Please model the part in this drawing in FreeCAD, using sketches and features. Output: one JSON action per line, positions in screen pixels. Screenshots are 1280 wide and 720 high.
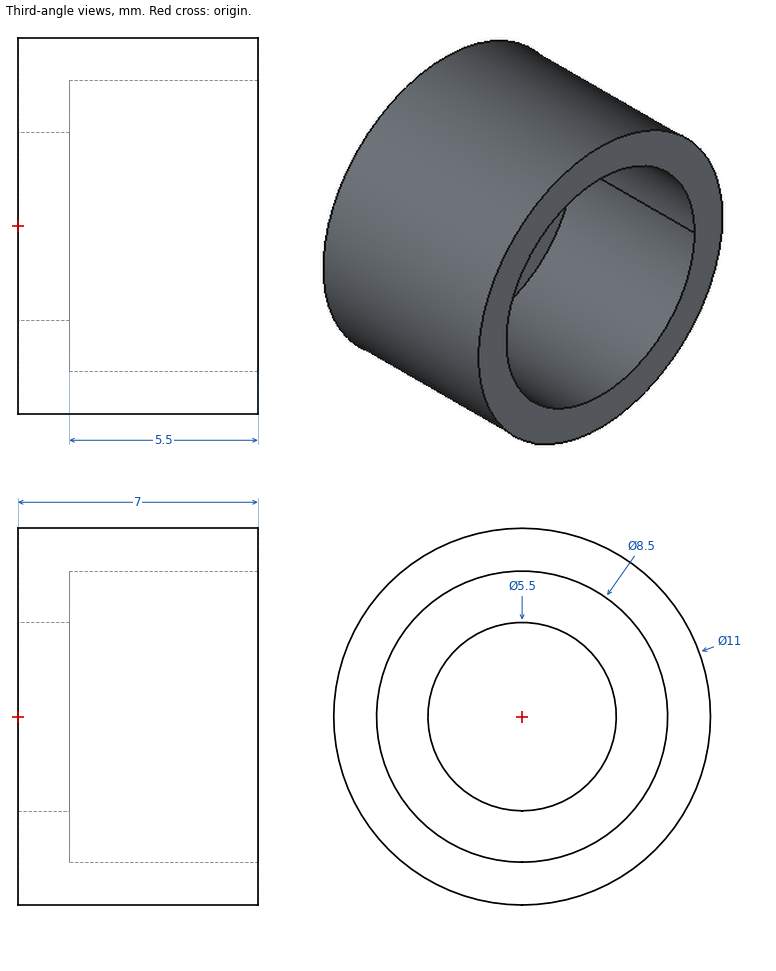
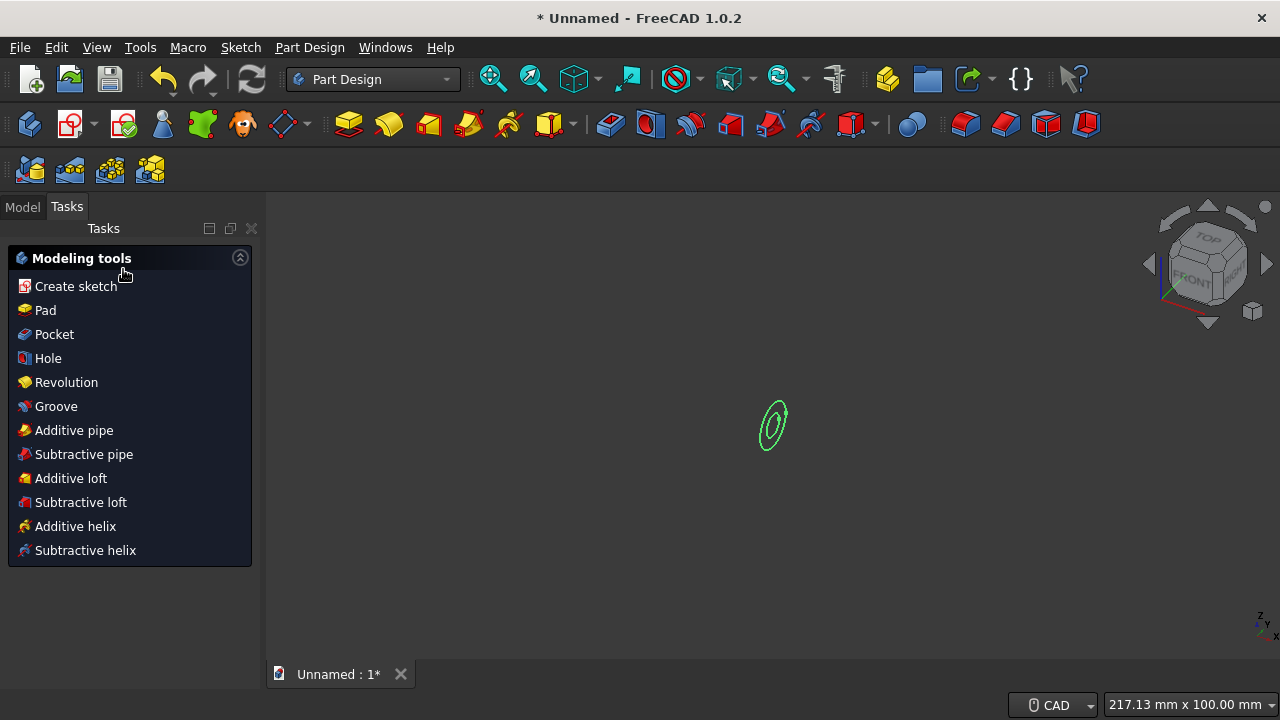
{"action": "left_click", "coordinate": [350, 124]}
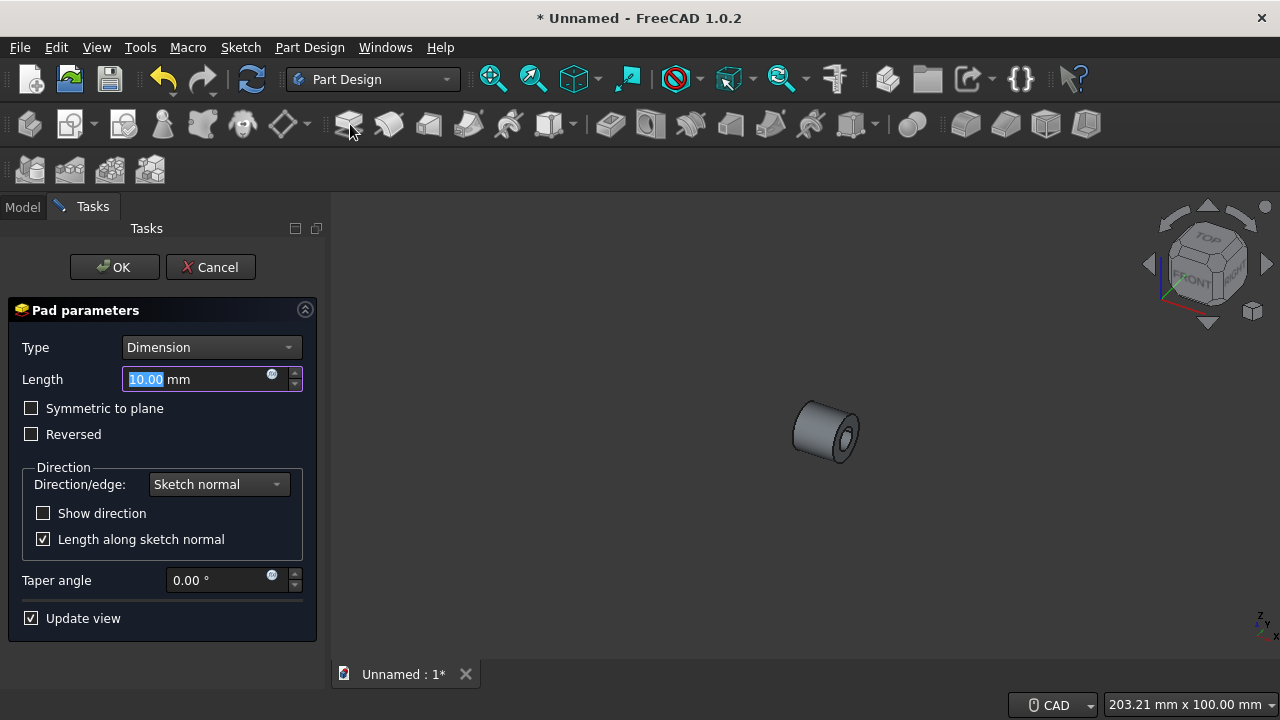
{"action": "type", "text": "7"}
{"action": "key", "text": "Tab"}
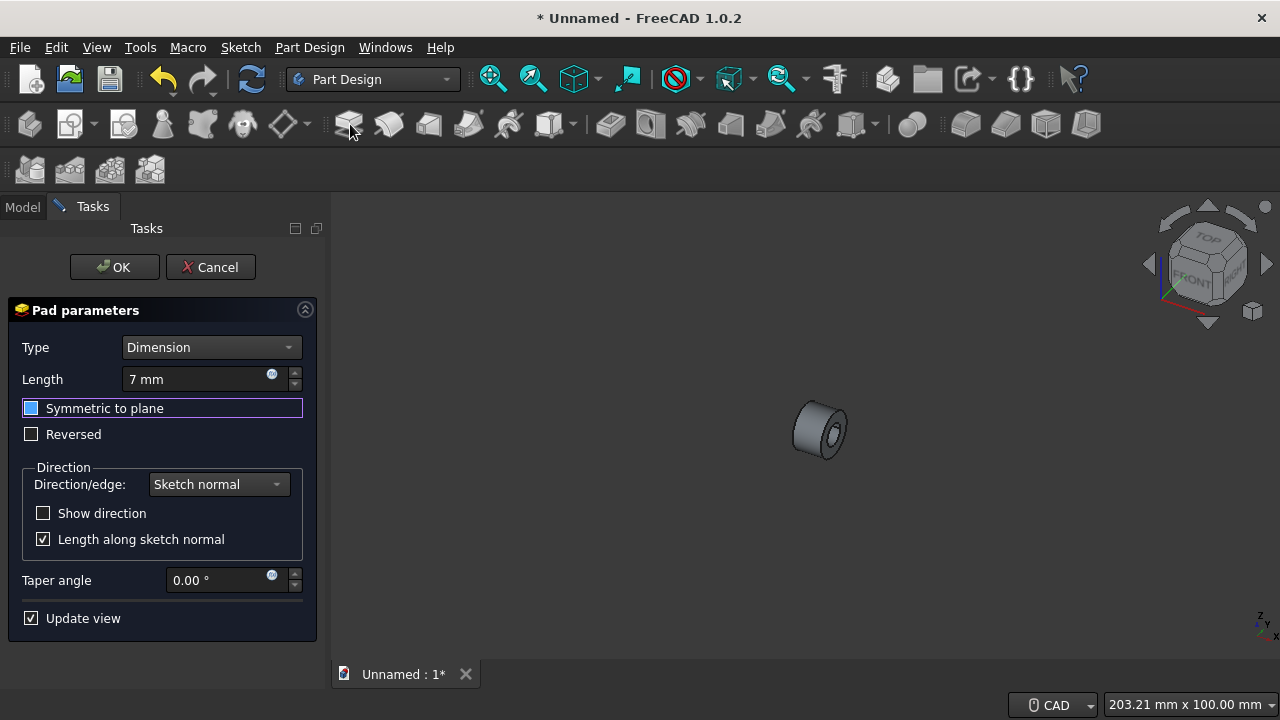
{"action": "left_click", "coordinate": [115, 267]}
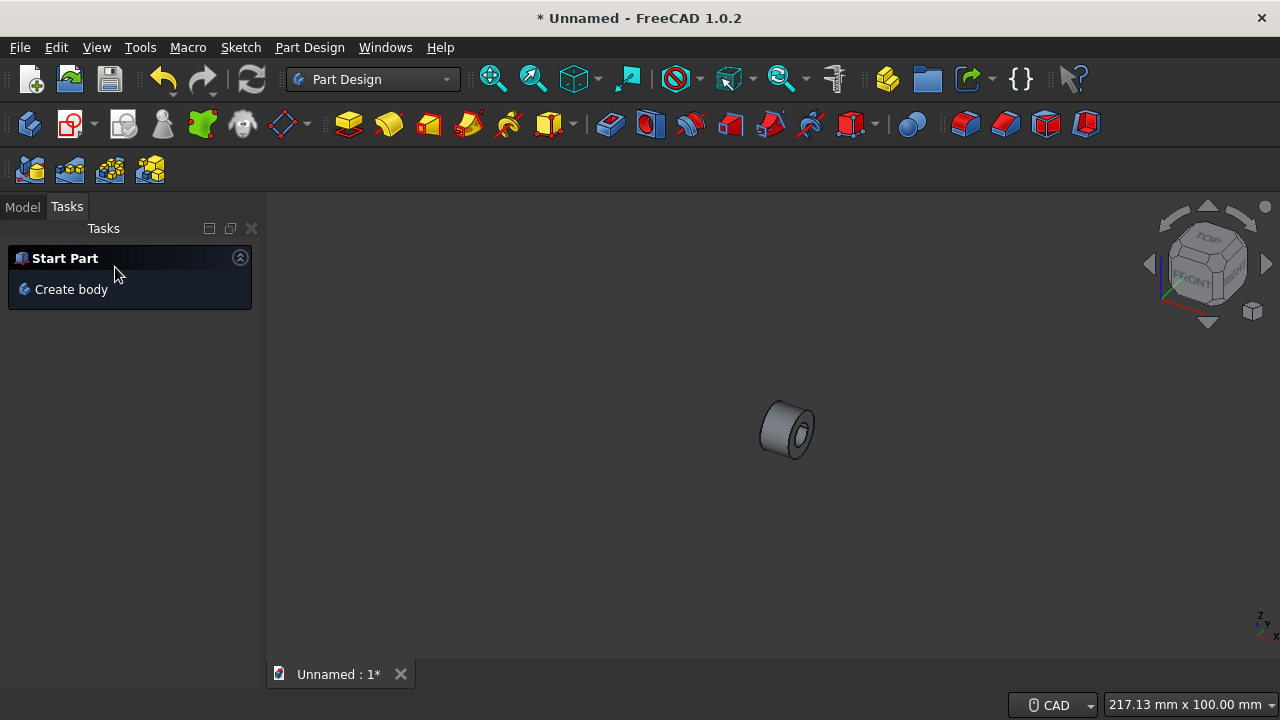
{"action": "left_click", "coordinate": [494, 80]}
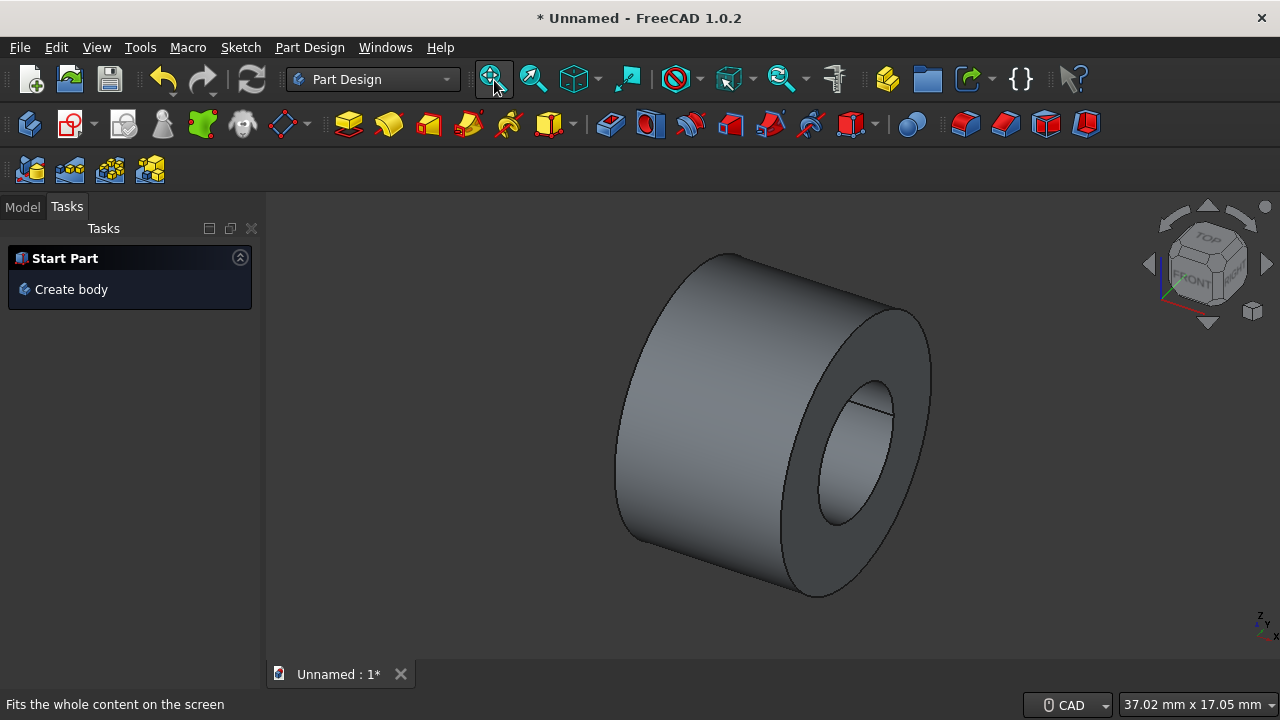
{"action": "left_click", "coordinate": [899, 480]}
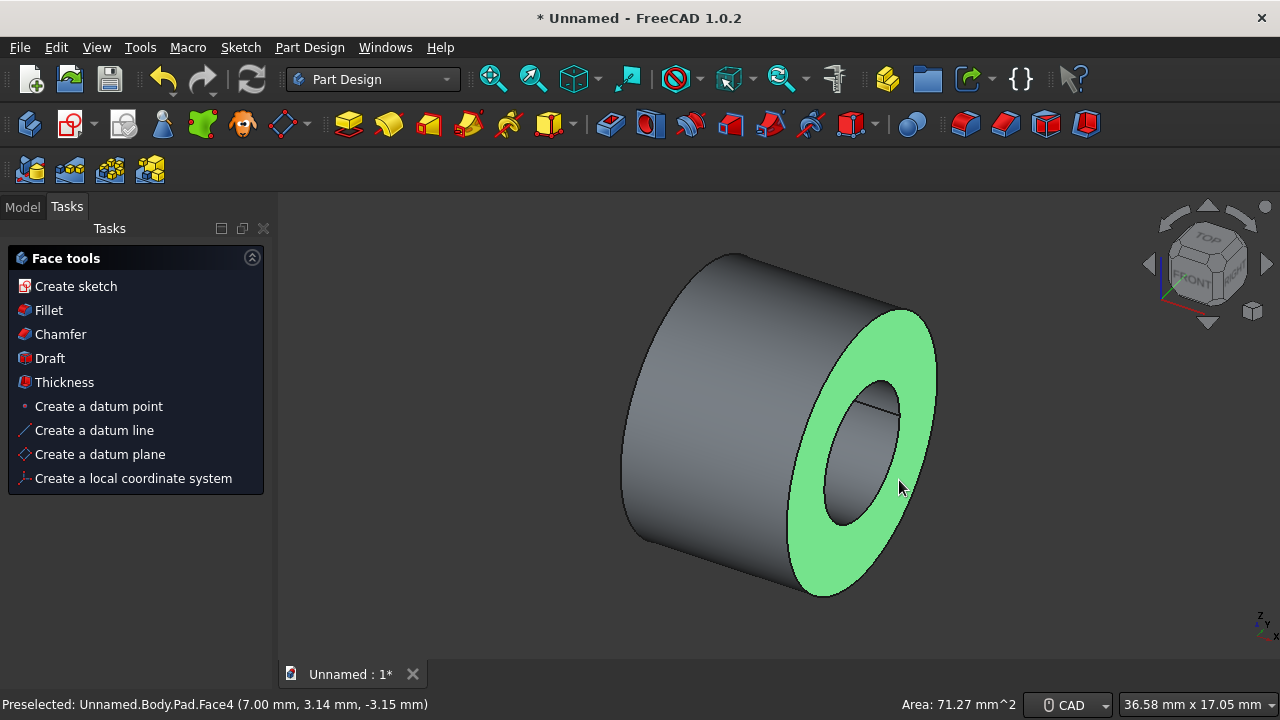
{"action": "left_click", "coordinate": [70, 124]}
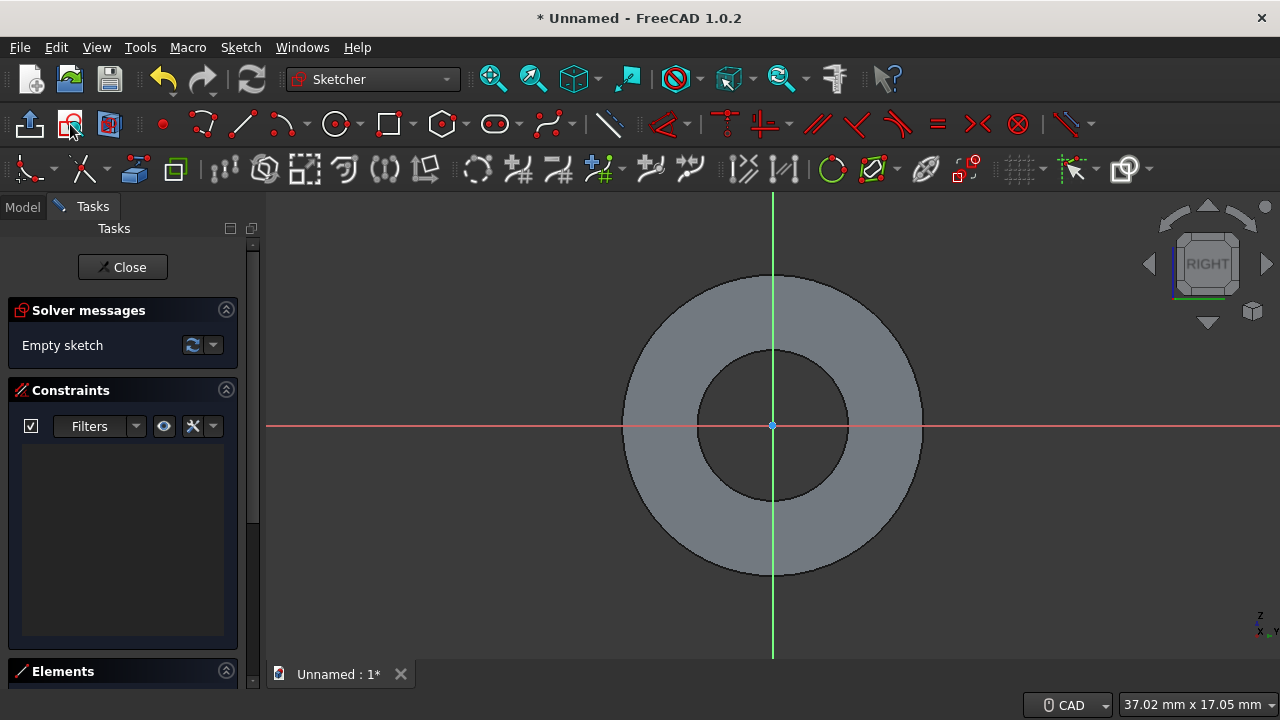
{"action": "left_click", "coordinate": [336, 124]}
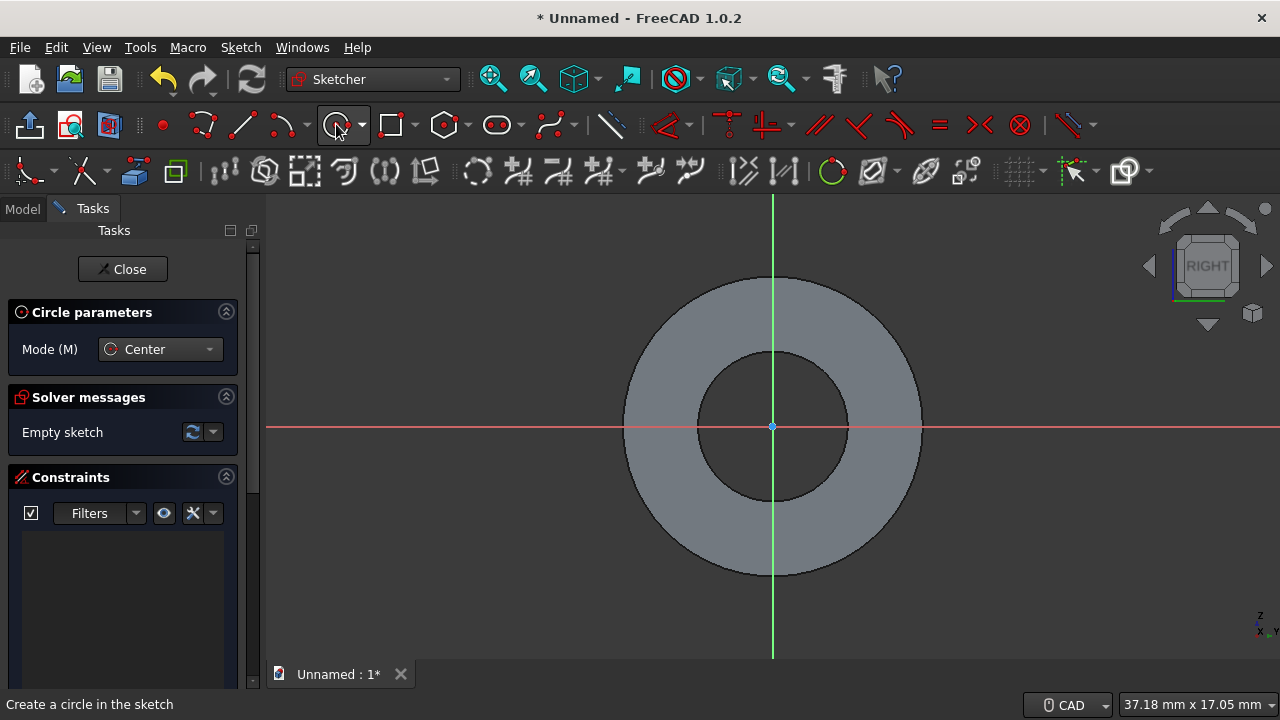
{"action": "left_click", "coordinate": [773, 426]}
{"action": "mouse_move", "coordinate": [855, 345]}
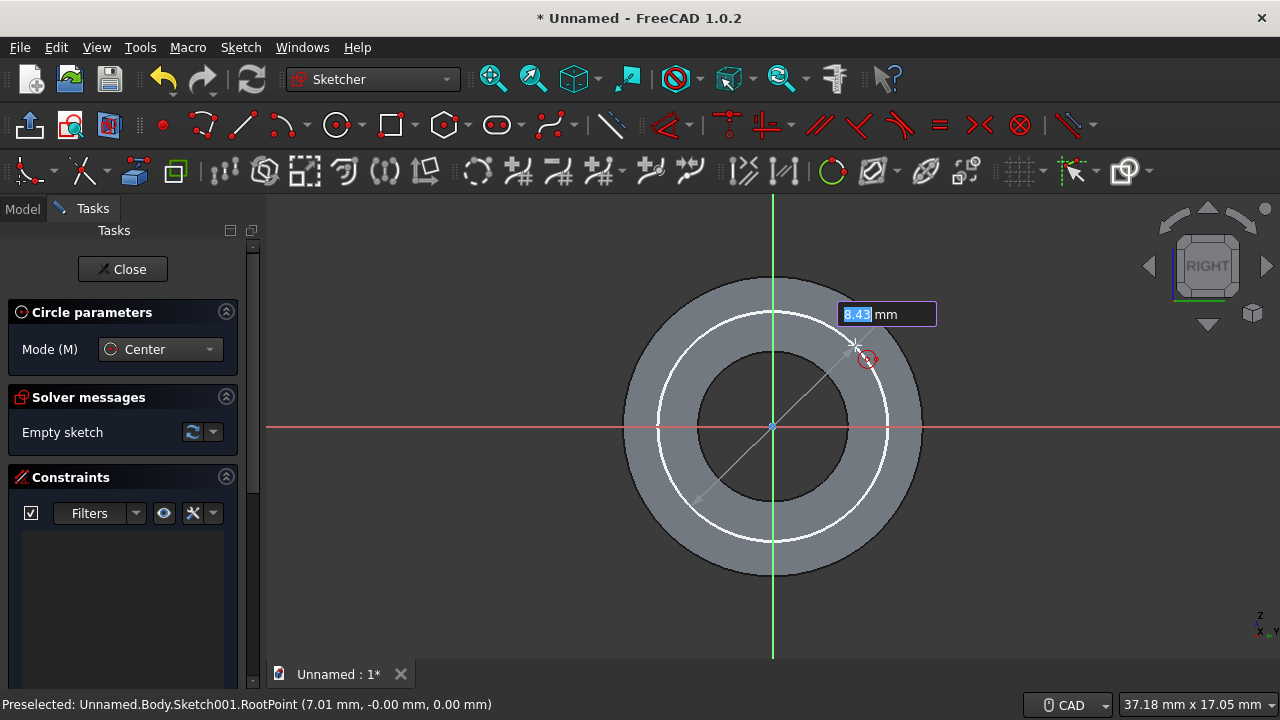
{"action": "type", "text": "8.5"}
{"action": "key", "text": "Return"}
{"action": "key", "text": "Escape"}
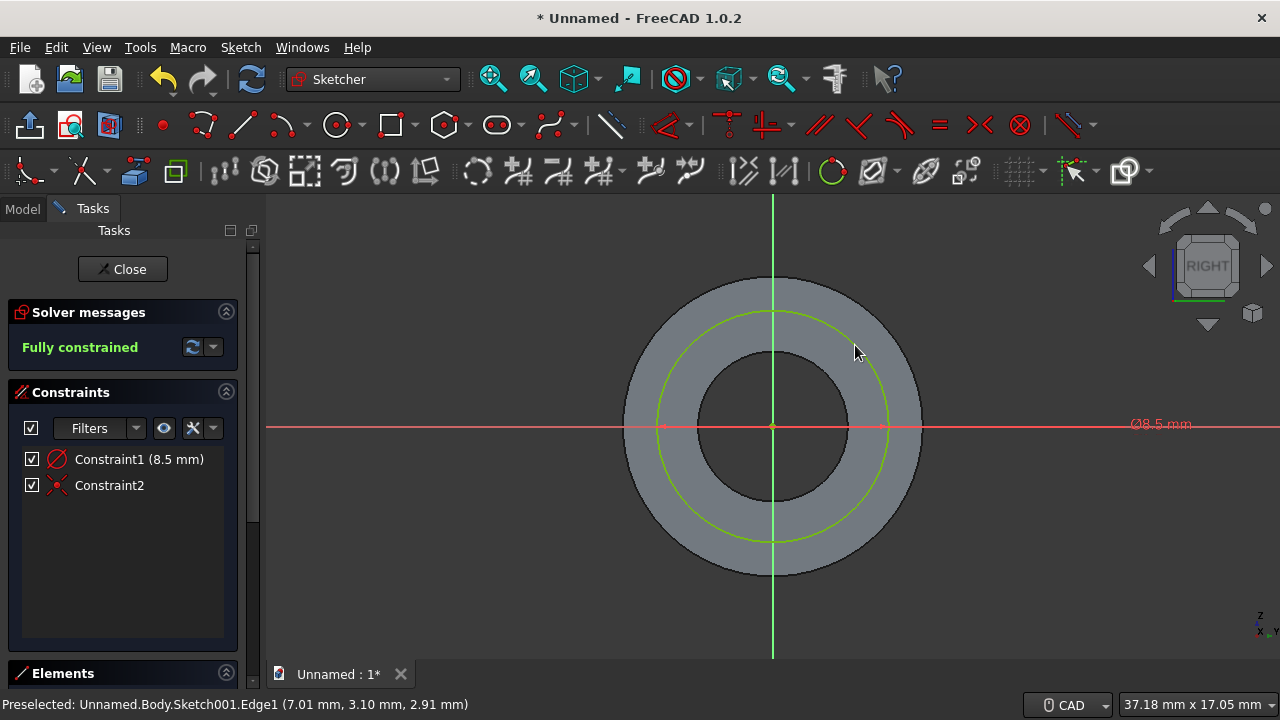
{"action": "left_click", "coordinate": [123, 269]}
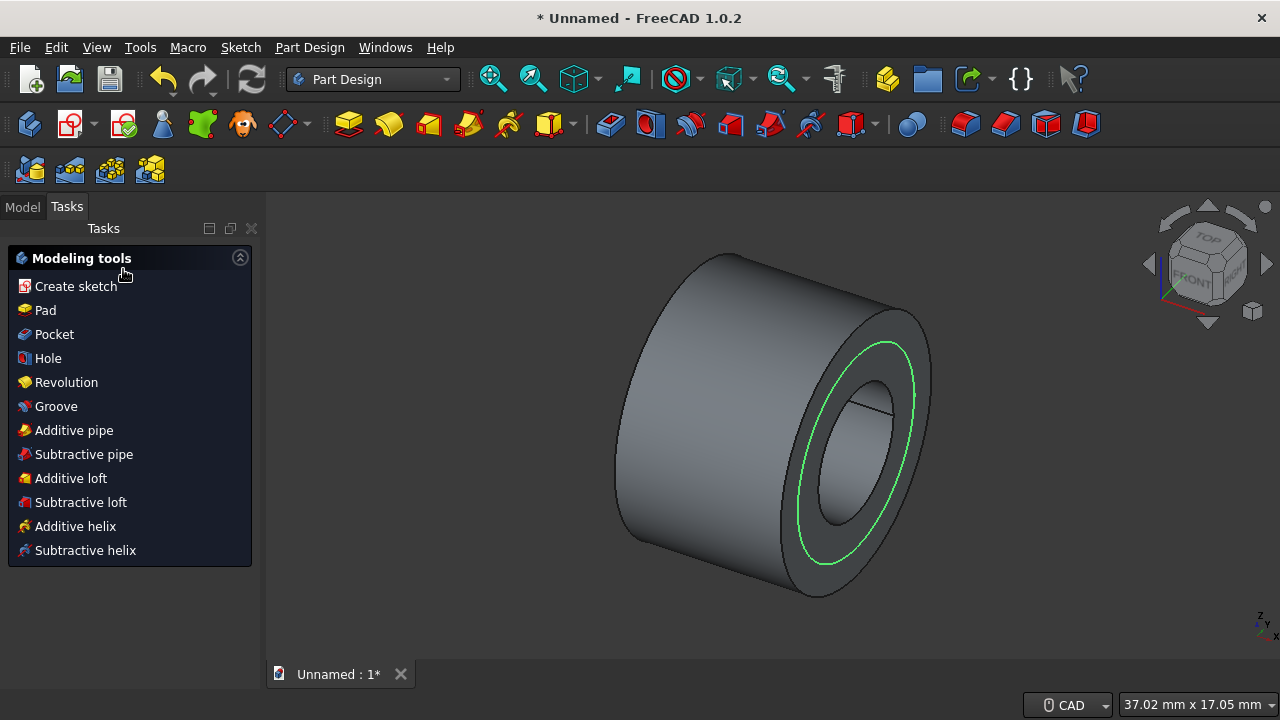
{"action": "left_click", "coordinate": [612, 124]}